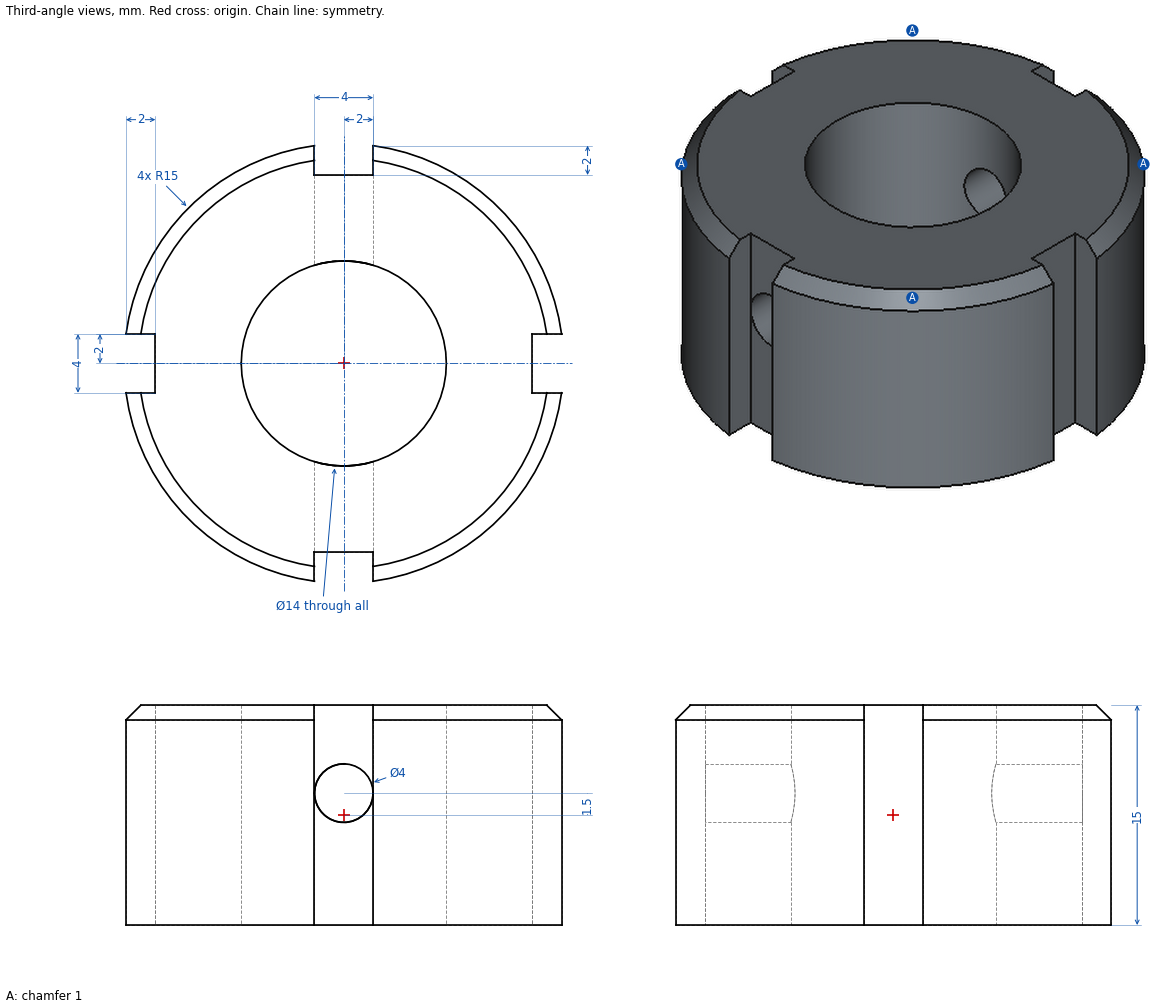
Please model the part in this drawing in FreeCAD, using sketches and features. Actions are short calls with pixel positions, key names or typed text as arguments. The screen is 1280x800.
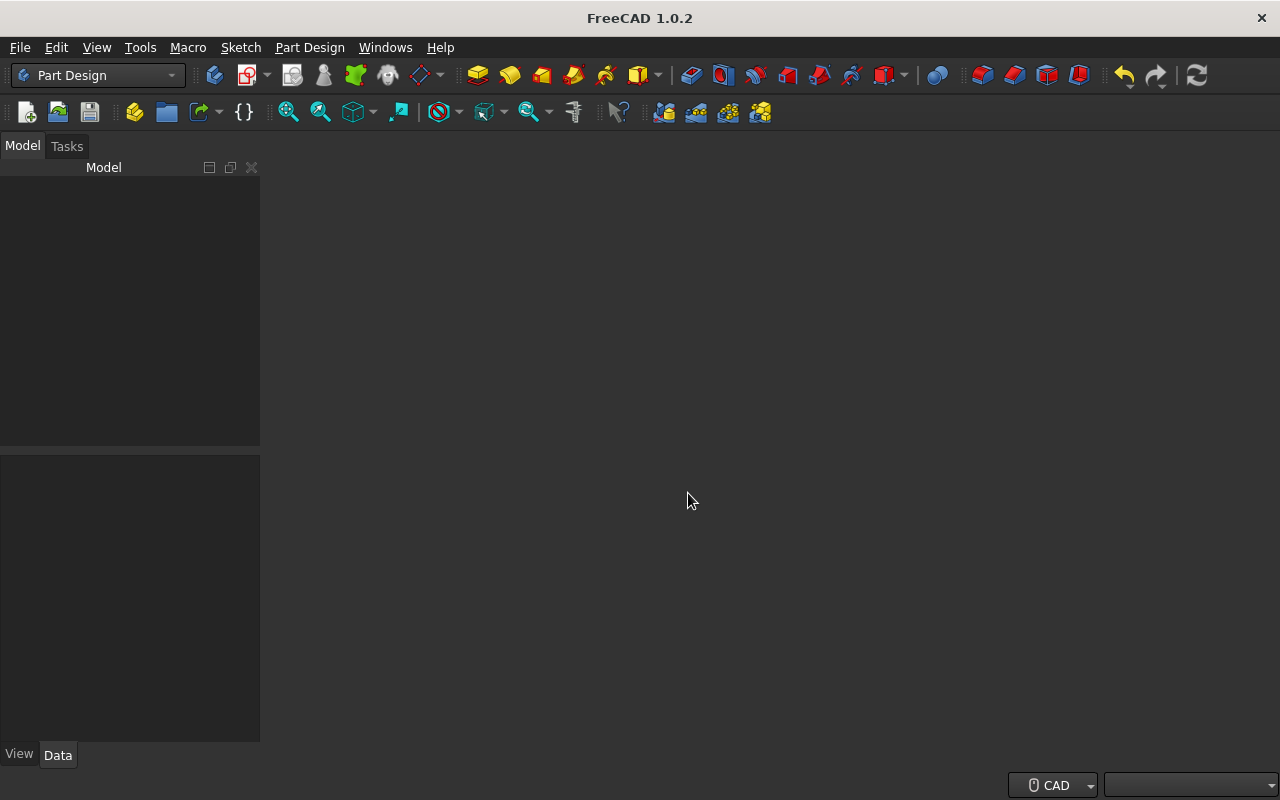
click(26, 112)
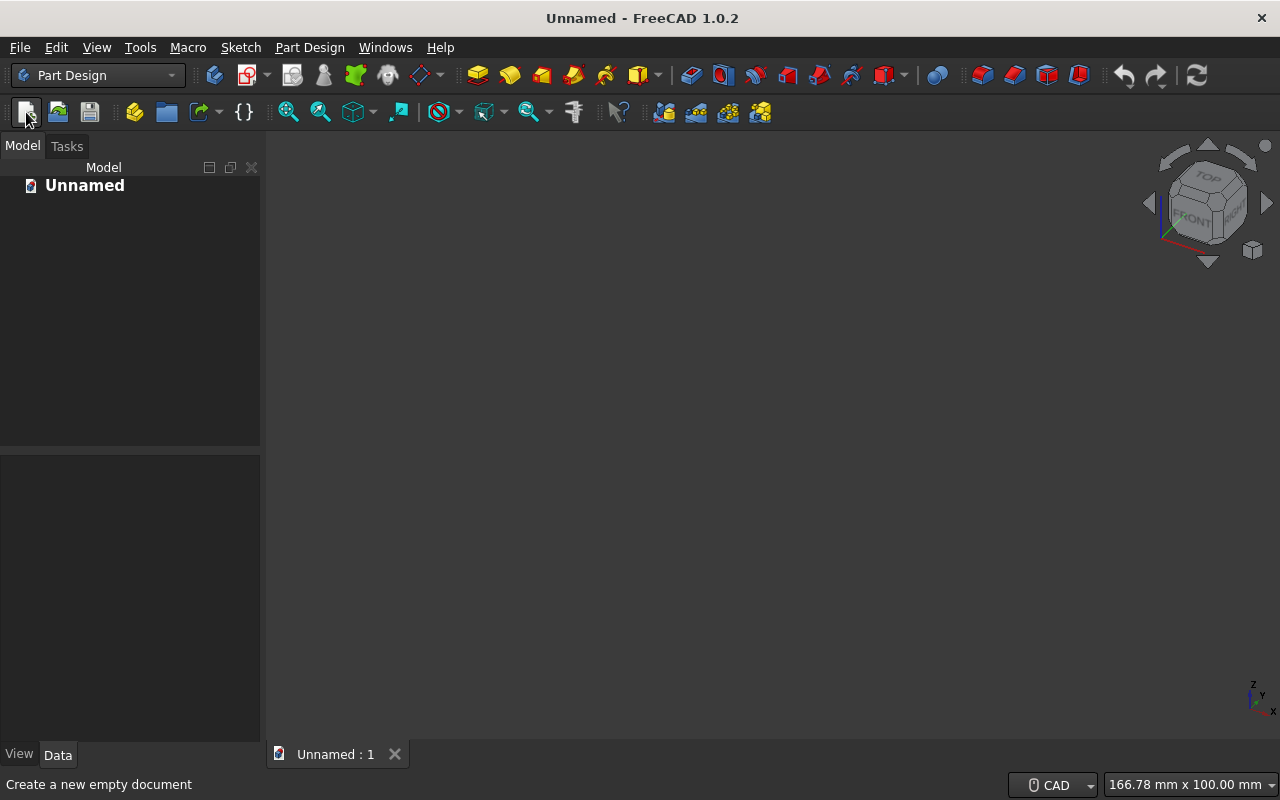
click(248, 76)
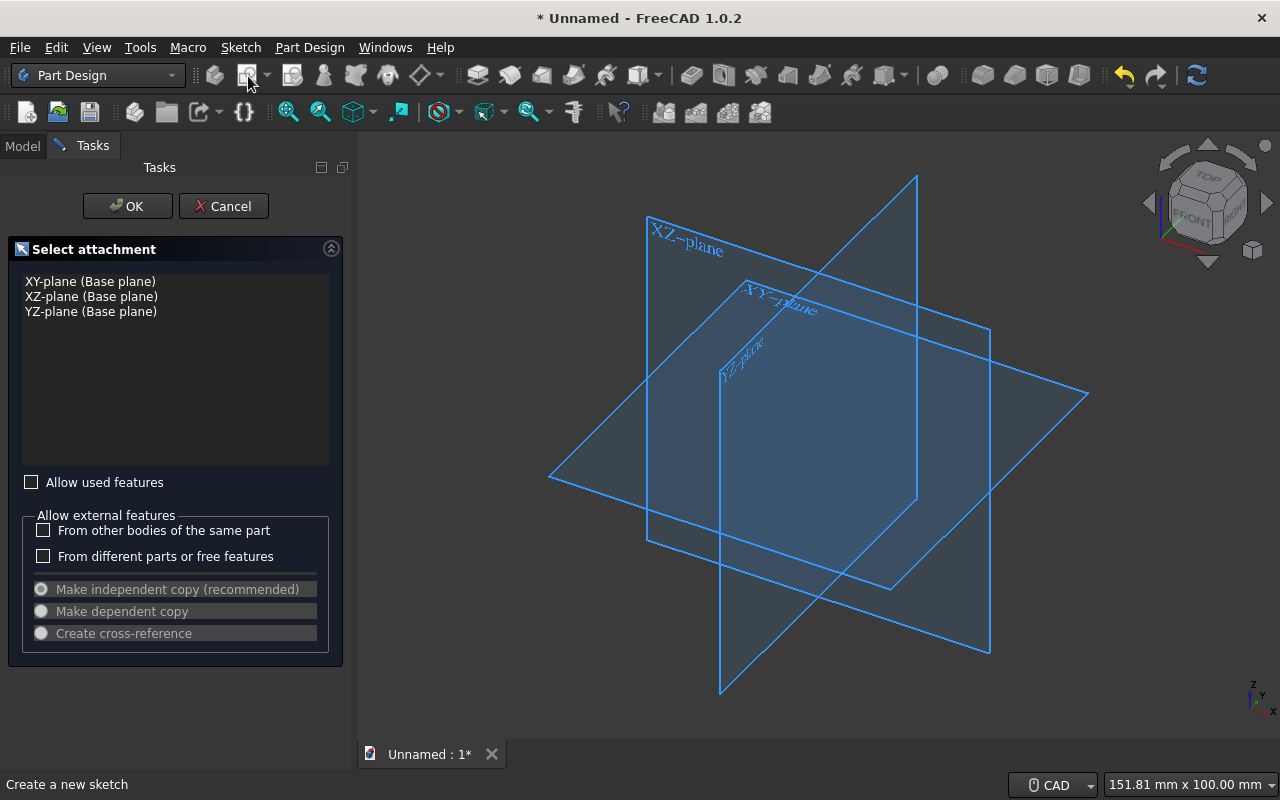
click(82, 282)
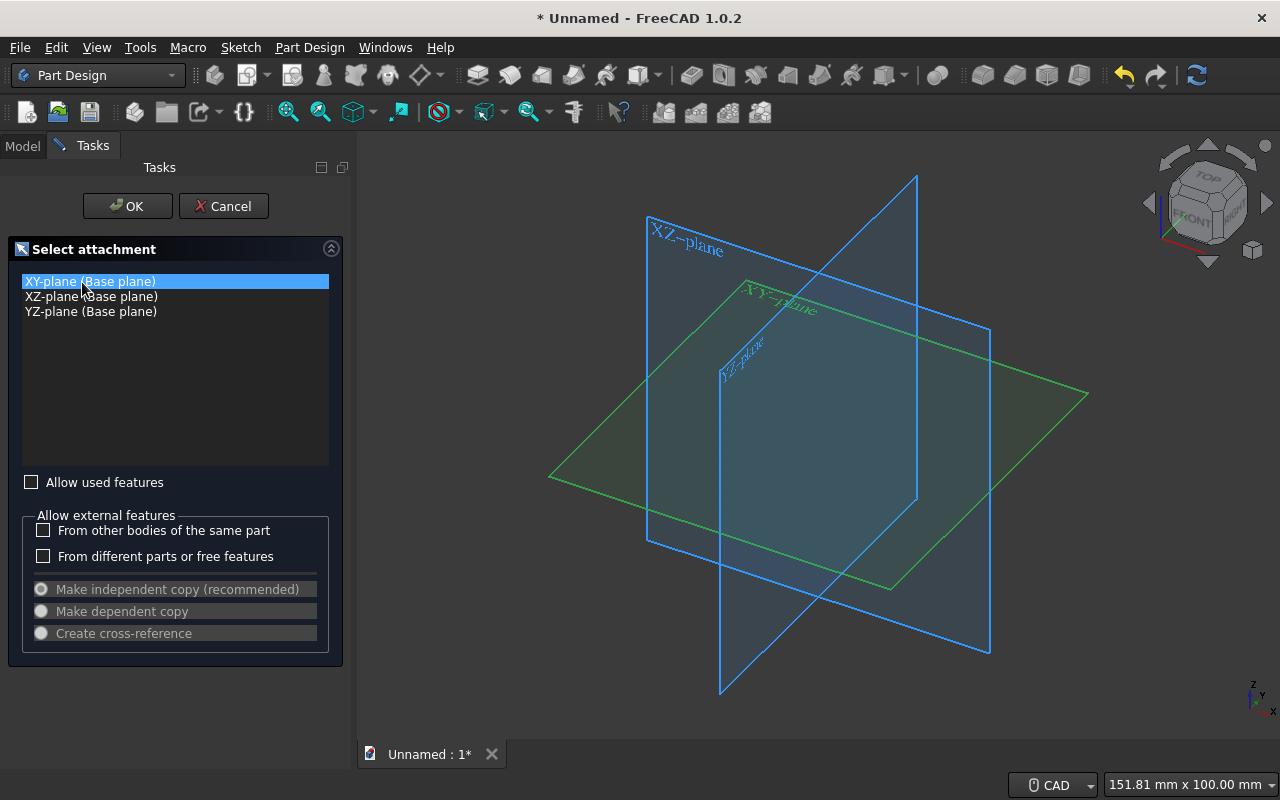
click(128, 206)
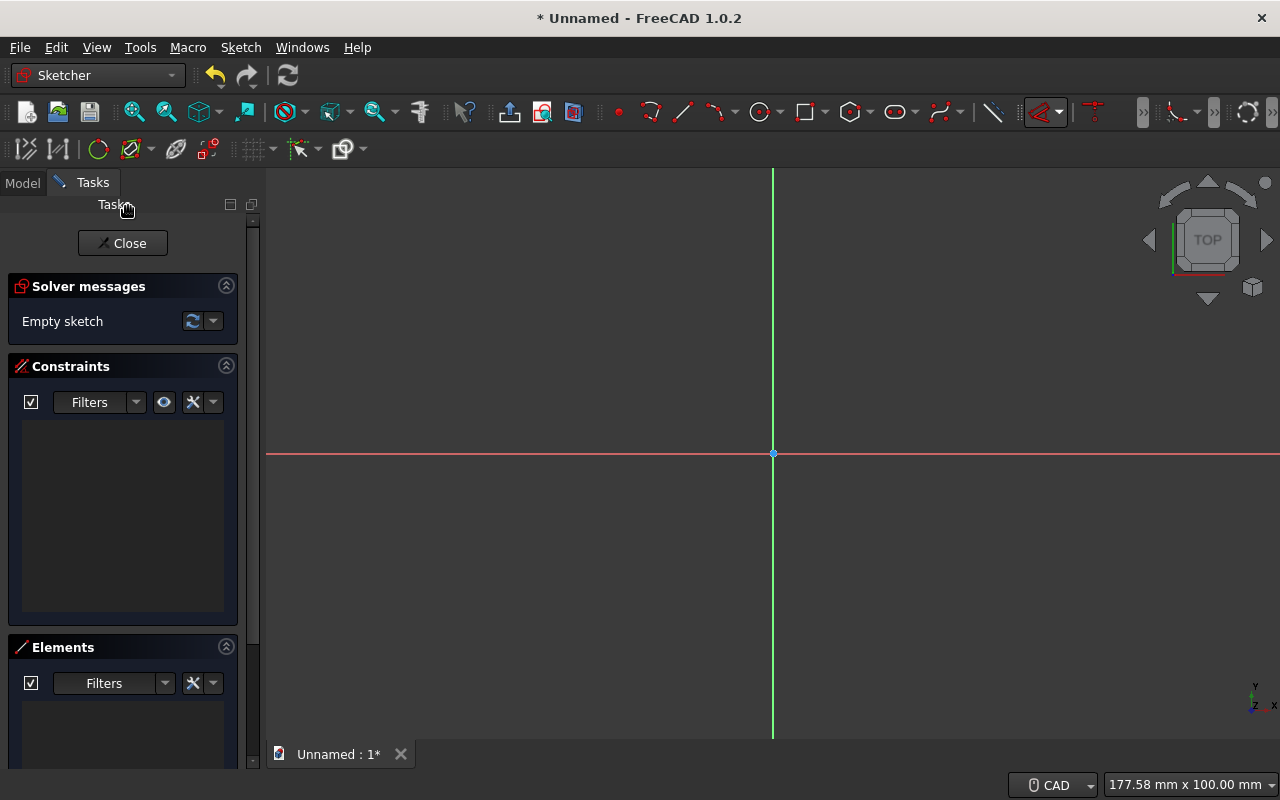
scroll(829, 454, up, 4)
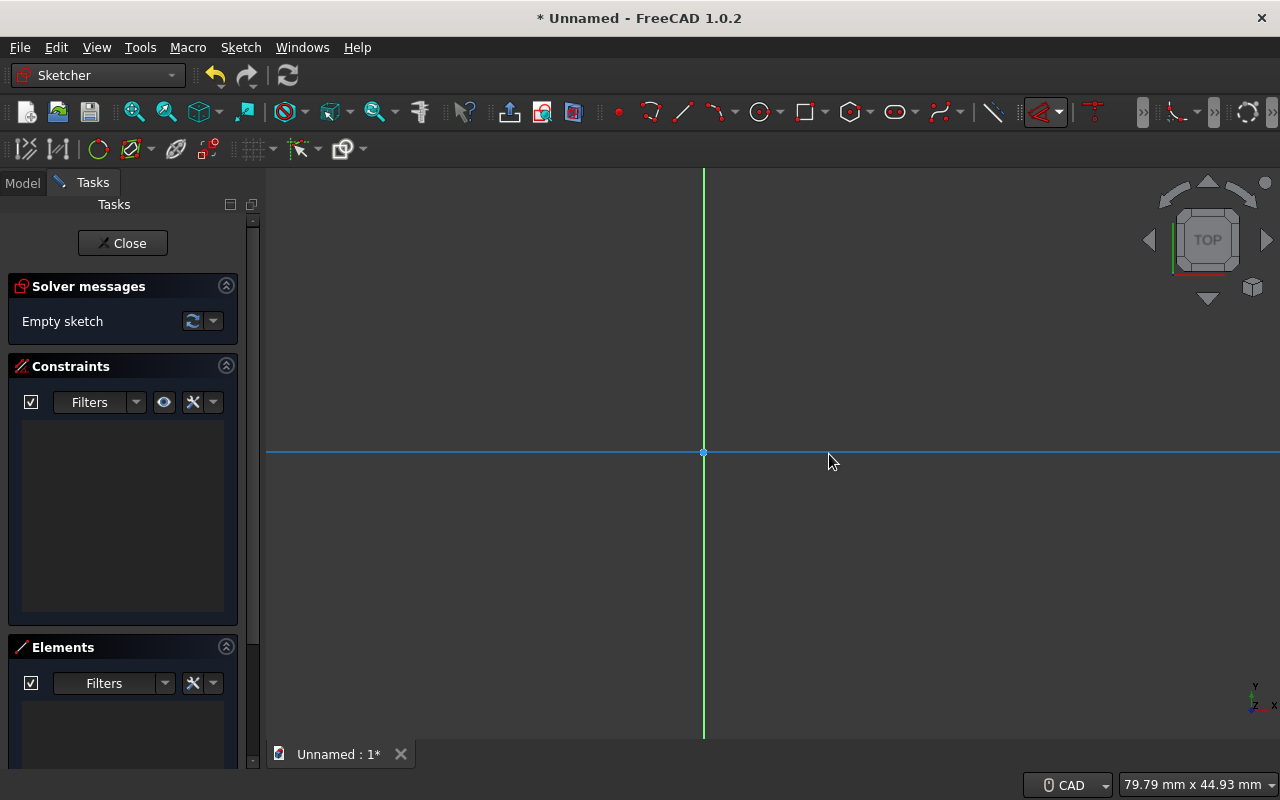
key(g)
key(m)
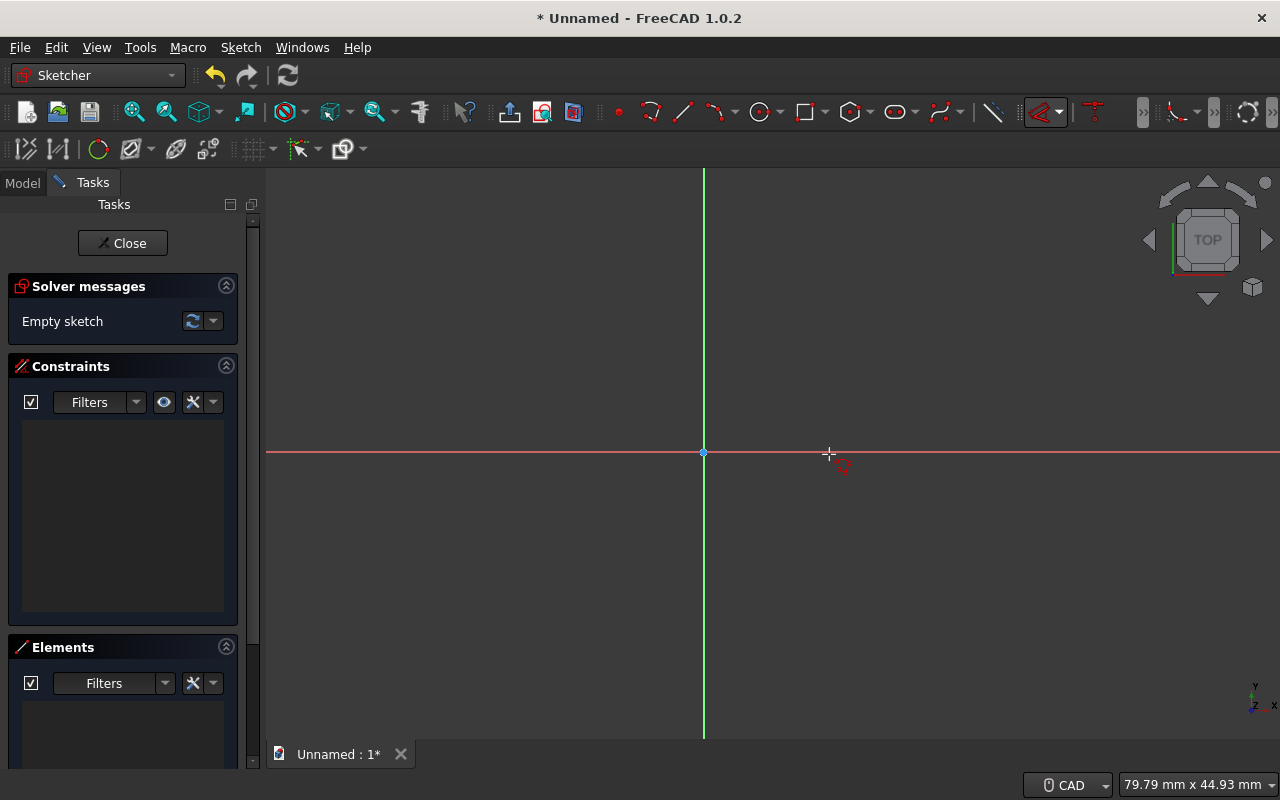
click(729, 263)
click(729, 289)
click(678, 289)
click(678, 263)
right_click(678, 263)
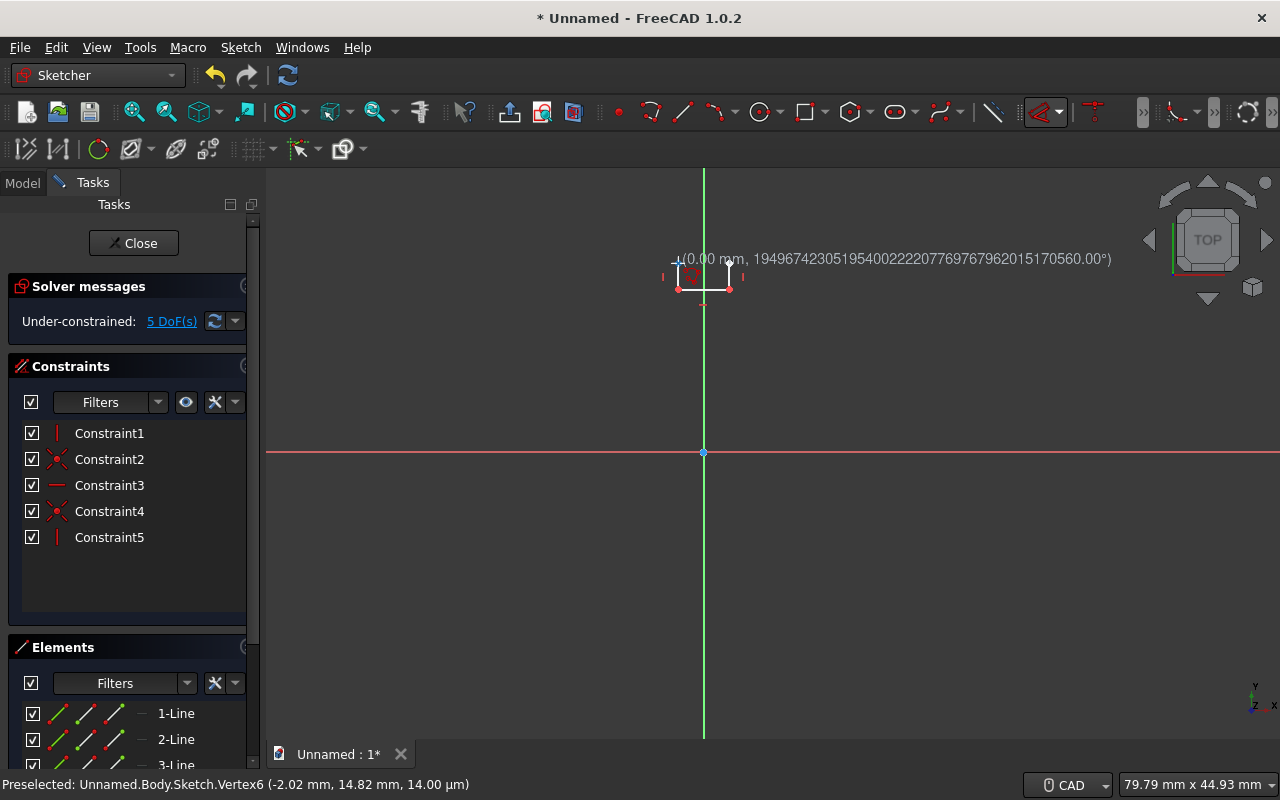
click(515, 427)
click(540, 427)
click(540, 478)
click(515, 478)
right_click(515, 478)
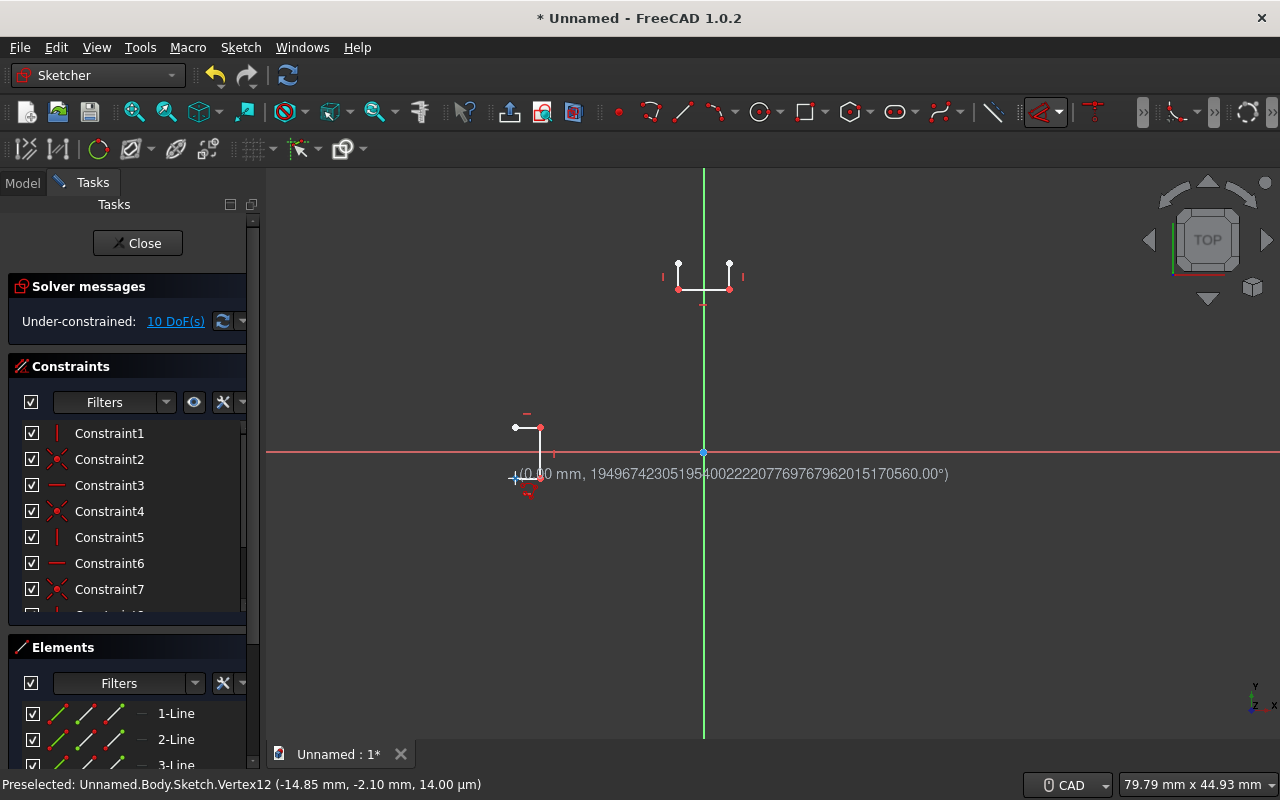
click(678, 641)
click(678, 616)
click(729, 616)
click(729, 641)
right_click(729, 641)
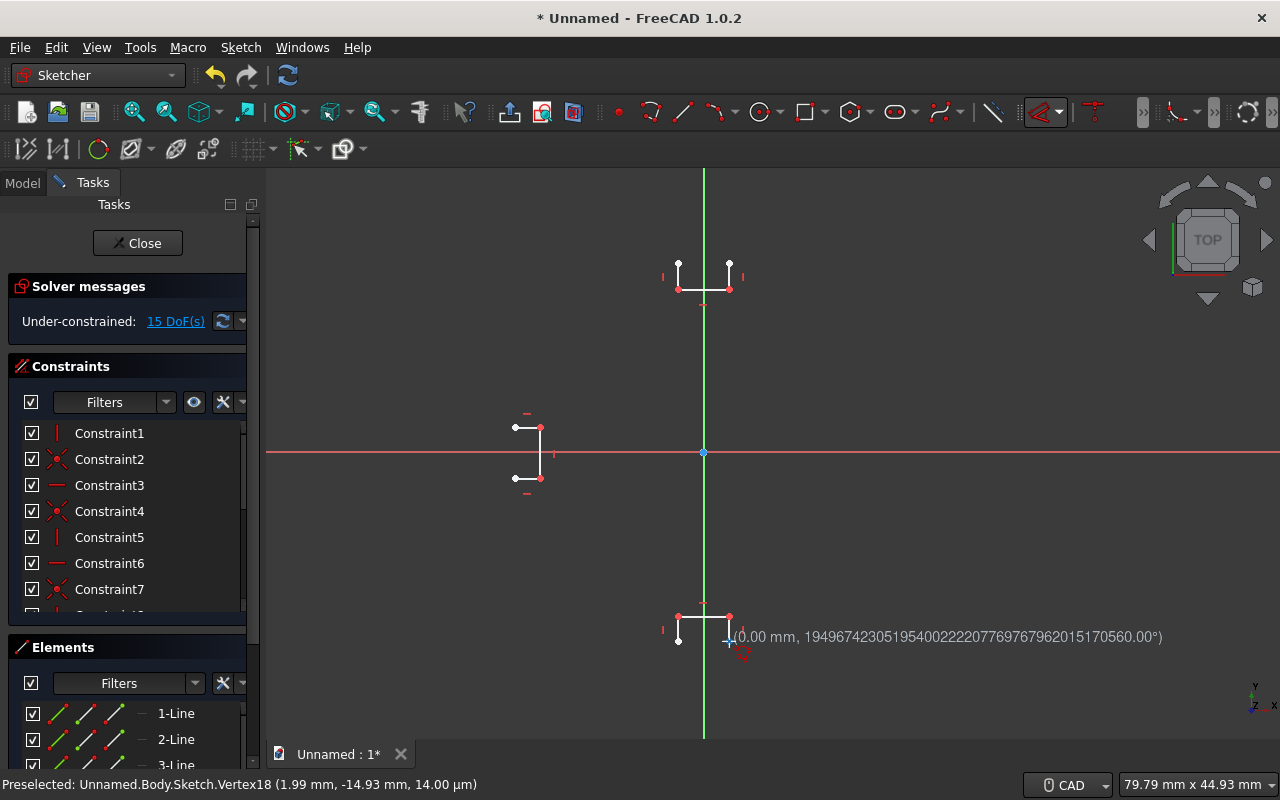
click(893, 478)
click(867, 478)
click(867, 427)
click(893, 427)
right_click(893, 427)